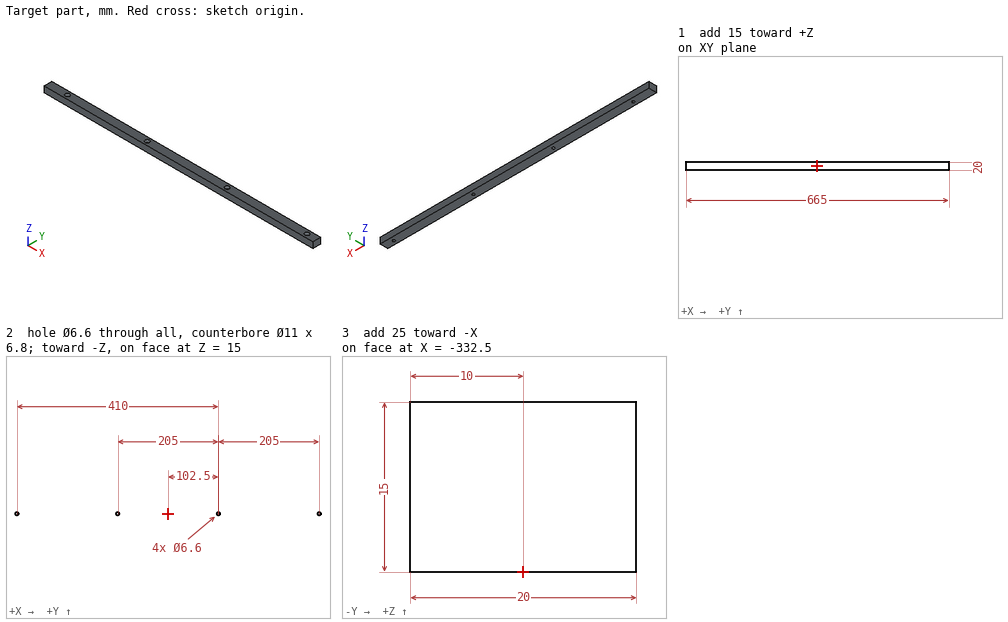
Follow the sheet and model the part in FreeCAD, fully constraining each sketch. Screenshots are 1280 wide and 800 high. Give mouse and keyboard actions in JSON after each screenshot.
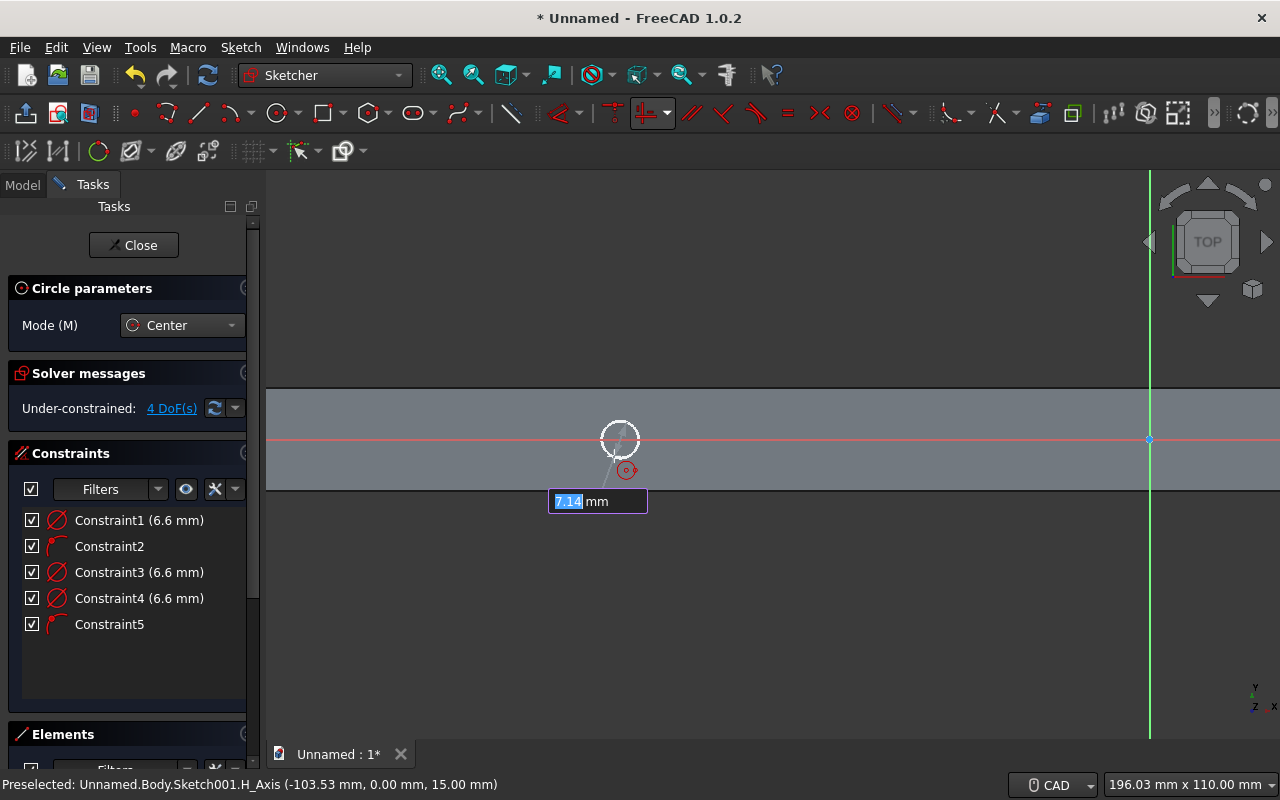
{"action": "type", "text": "6.6"}
{"action": "key", "text": "Return"}
{"action": "key", "text": "Escape"}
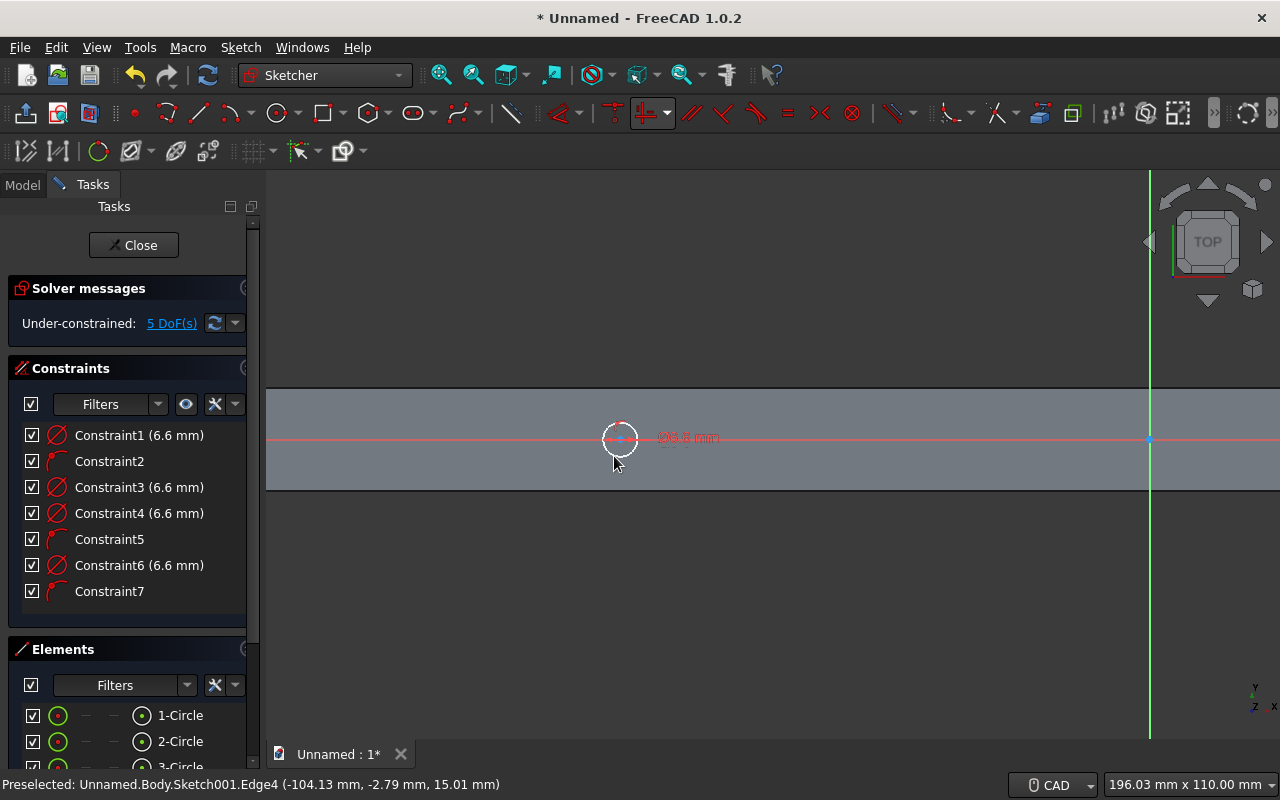
{"action": "scroll", "coordinate": [616, 457], "scroll_direction": "down", "scroll_amount": 9}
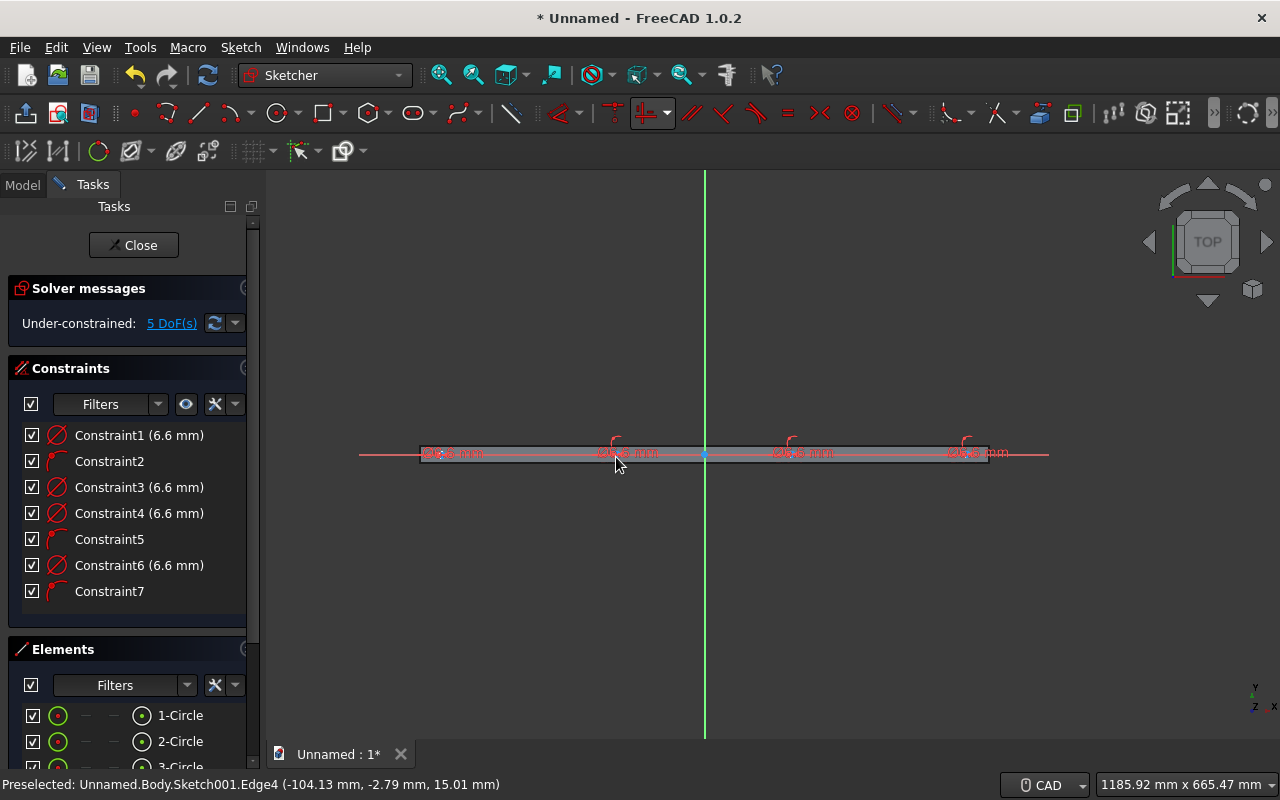
{"action": "left_click", "coordinate": [442, 455]}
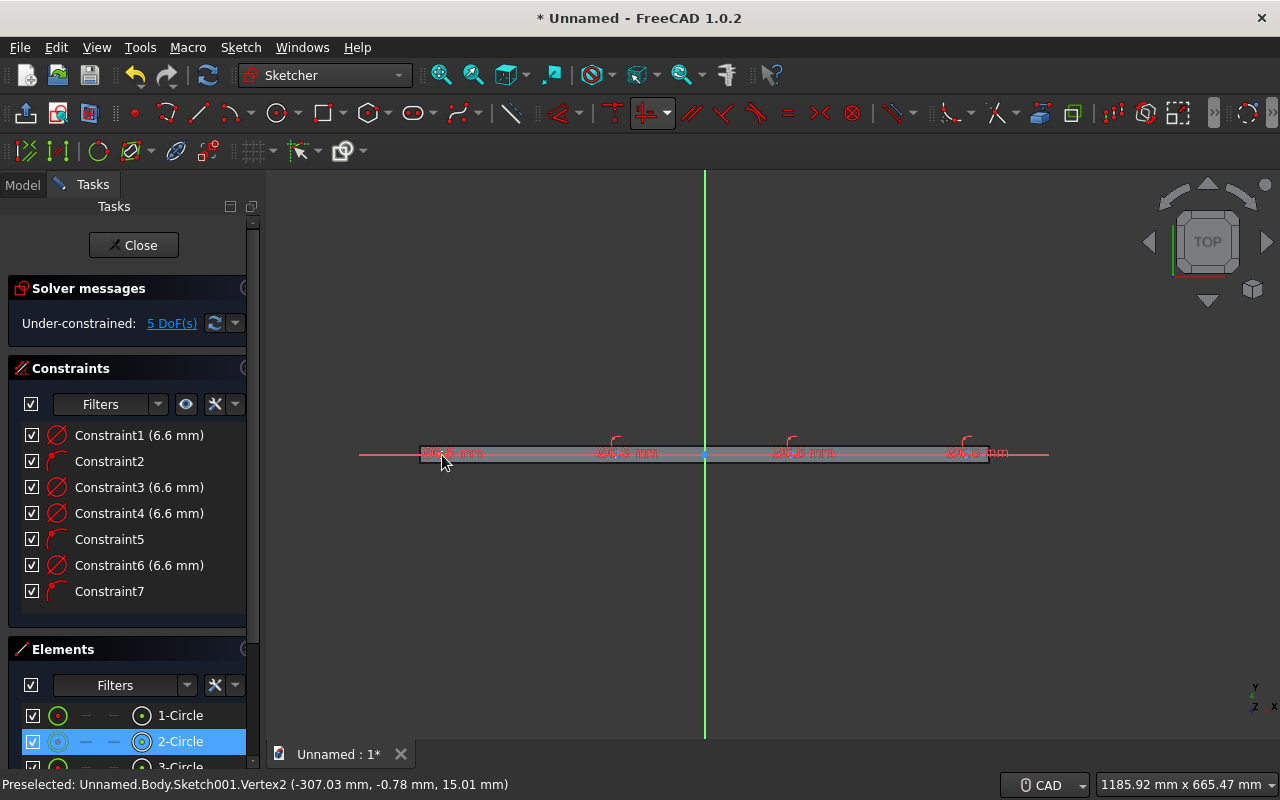
{"action": "left_click", "coordinate": [529, 455]}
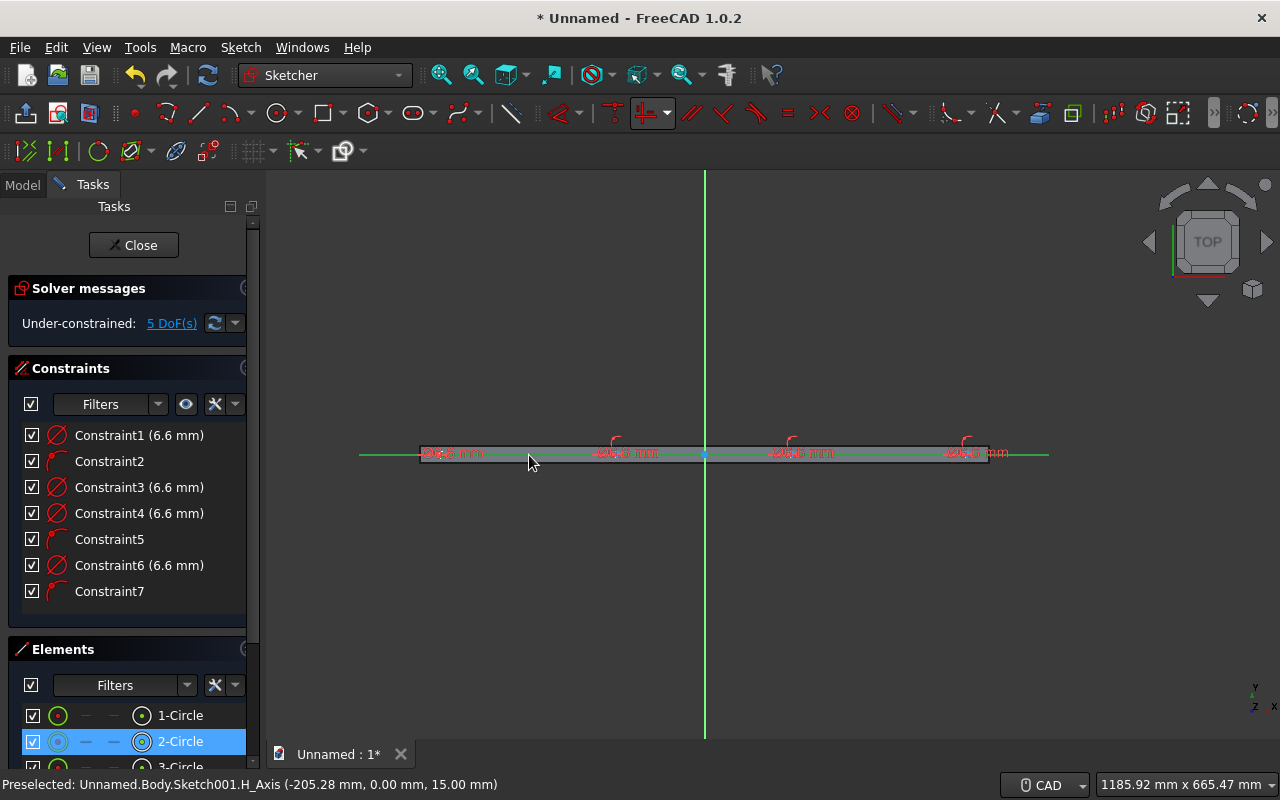
{"action": "key", "text": "c"}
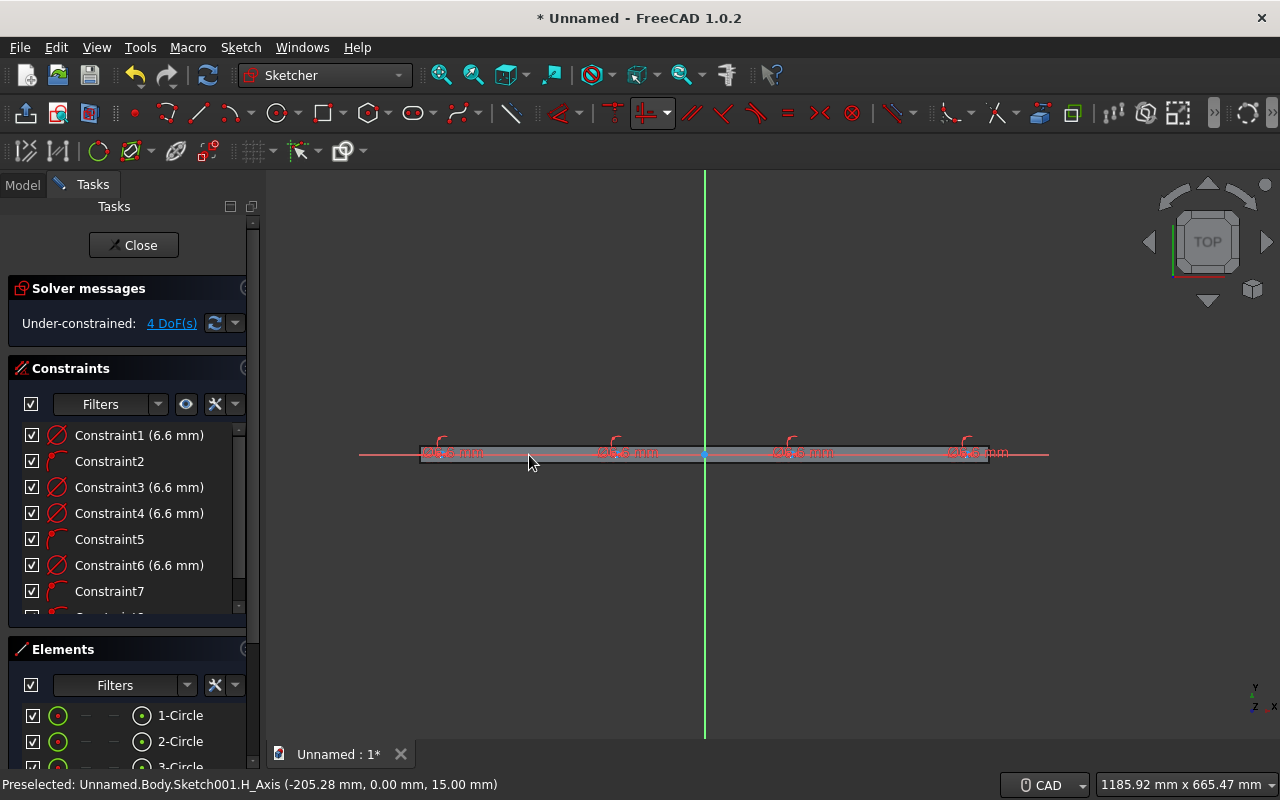
{"action": "left_click", "coordinate": [792, 455]}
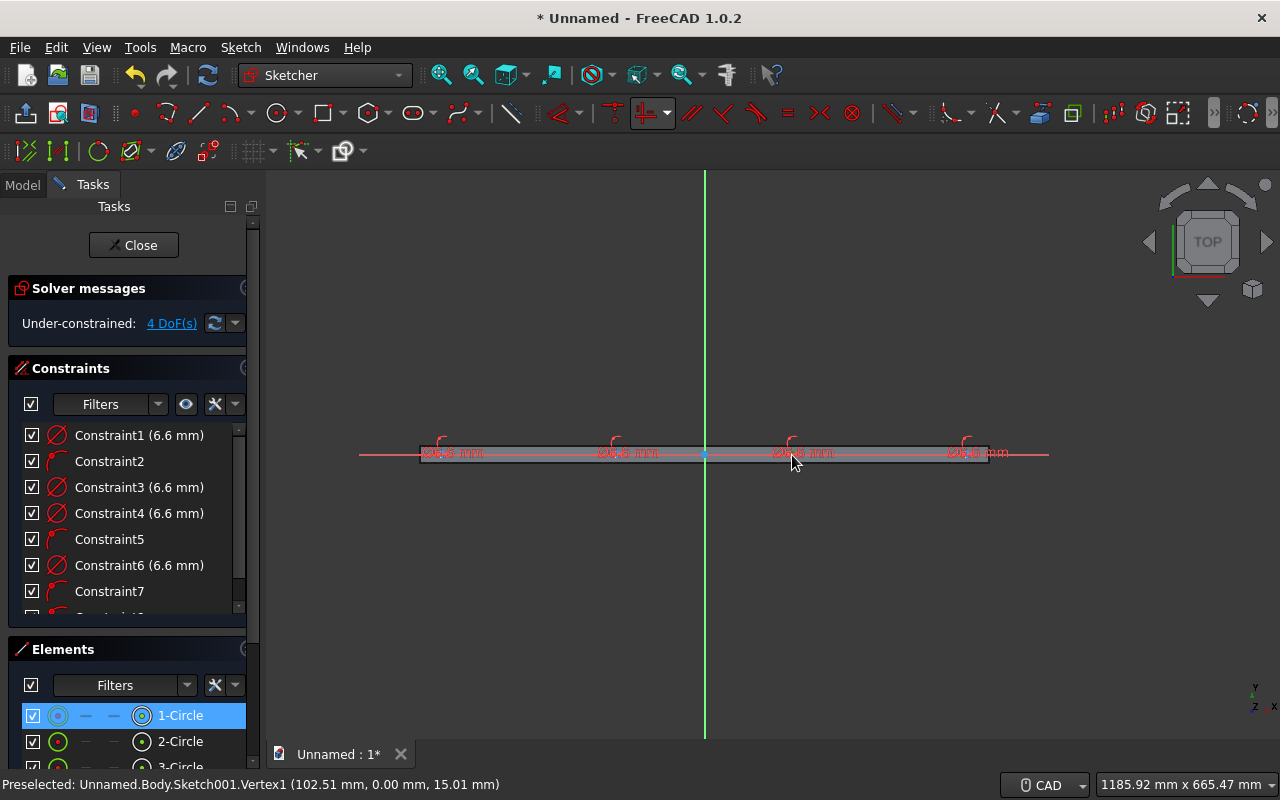
{"action": "left_click", "coordinate": [442, 455]}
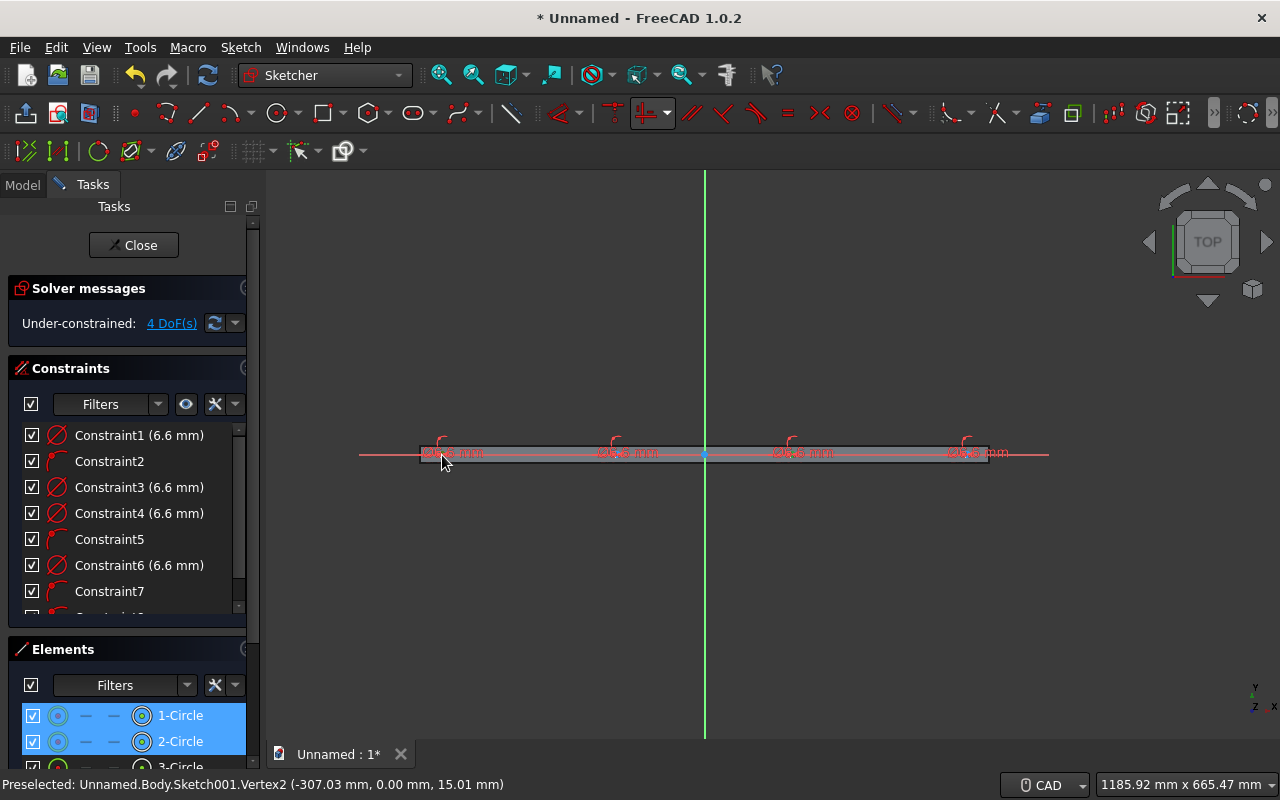
{"action": "key", "text": "l"}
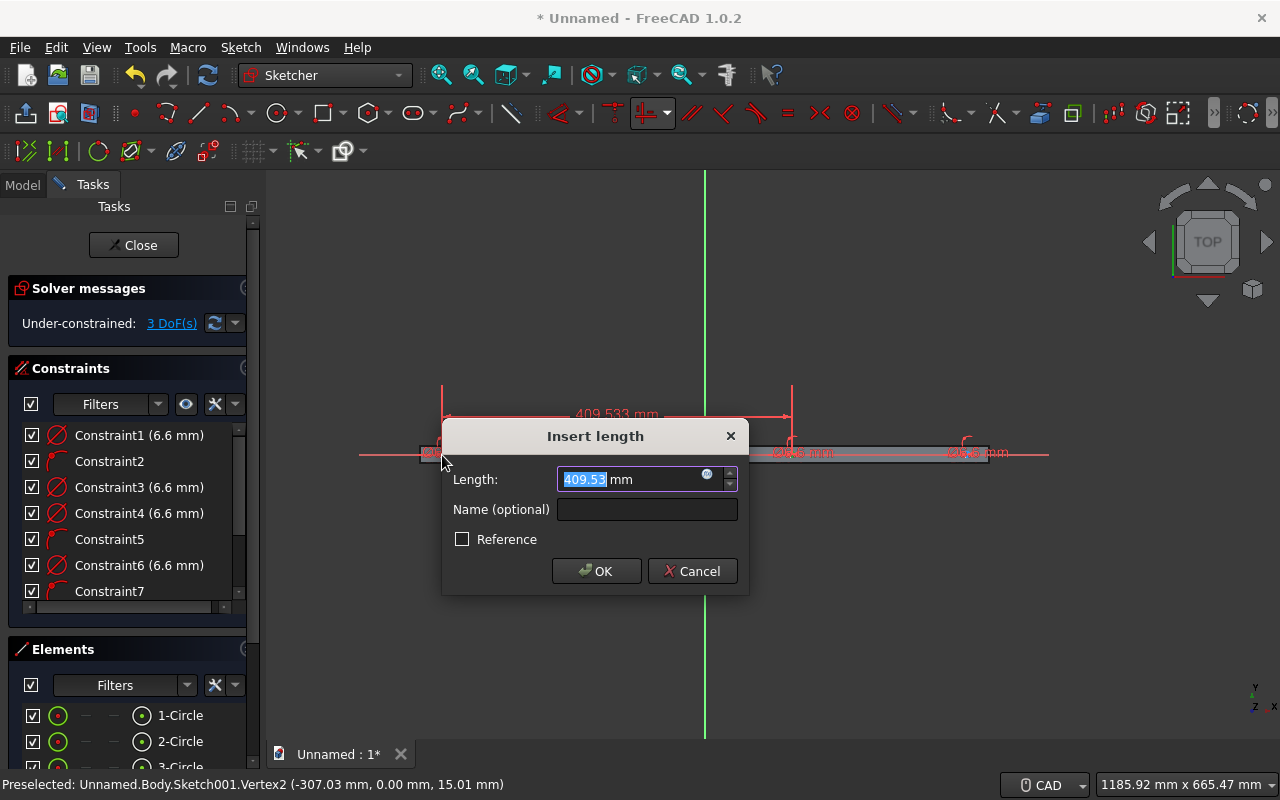
{"action": "type", "text": "410"}
{"action": "key", "text": "Return"}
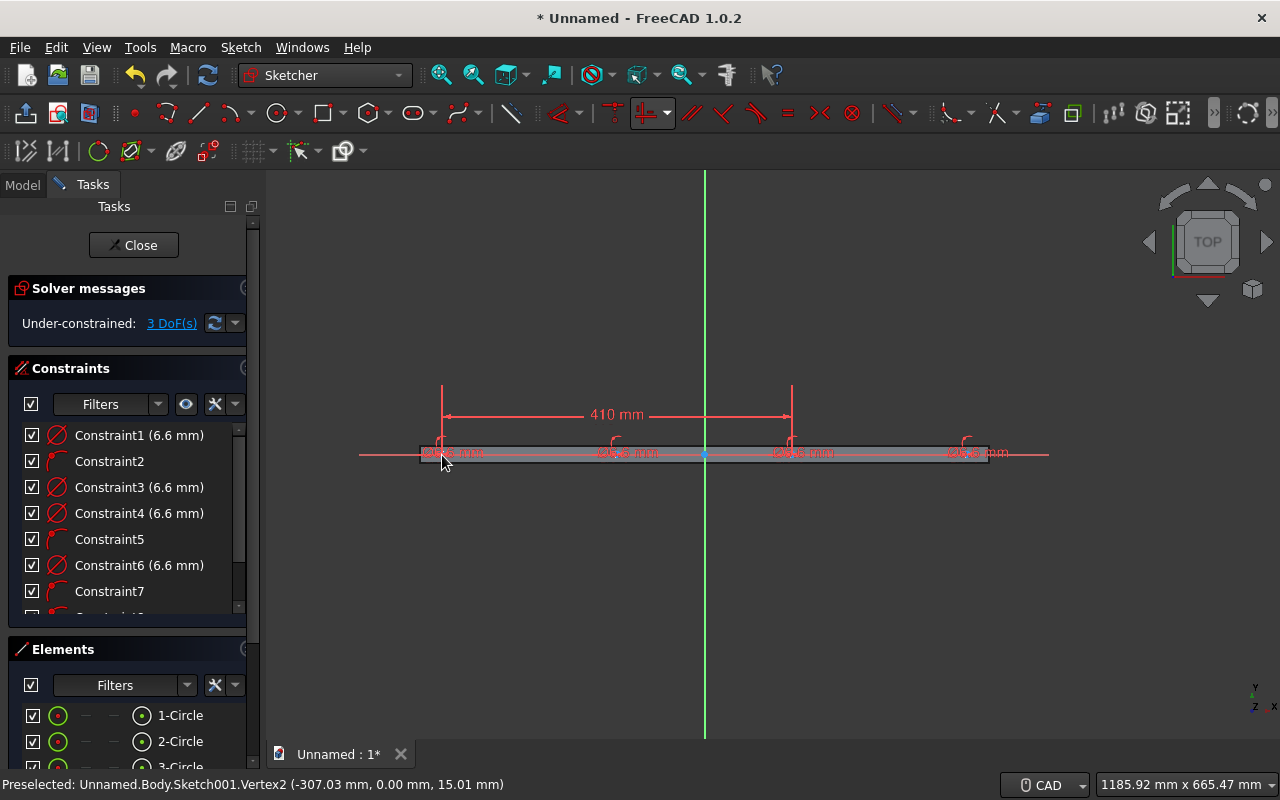
{"action": "left_click", "coordinate": [792, 455]}